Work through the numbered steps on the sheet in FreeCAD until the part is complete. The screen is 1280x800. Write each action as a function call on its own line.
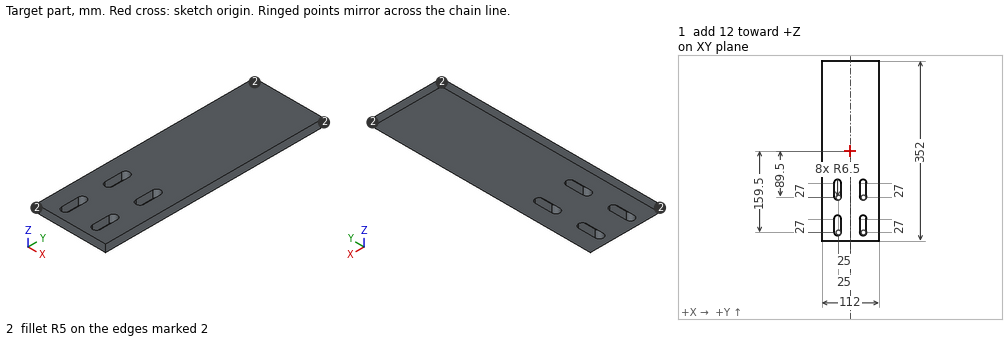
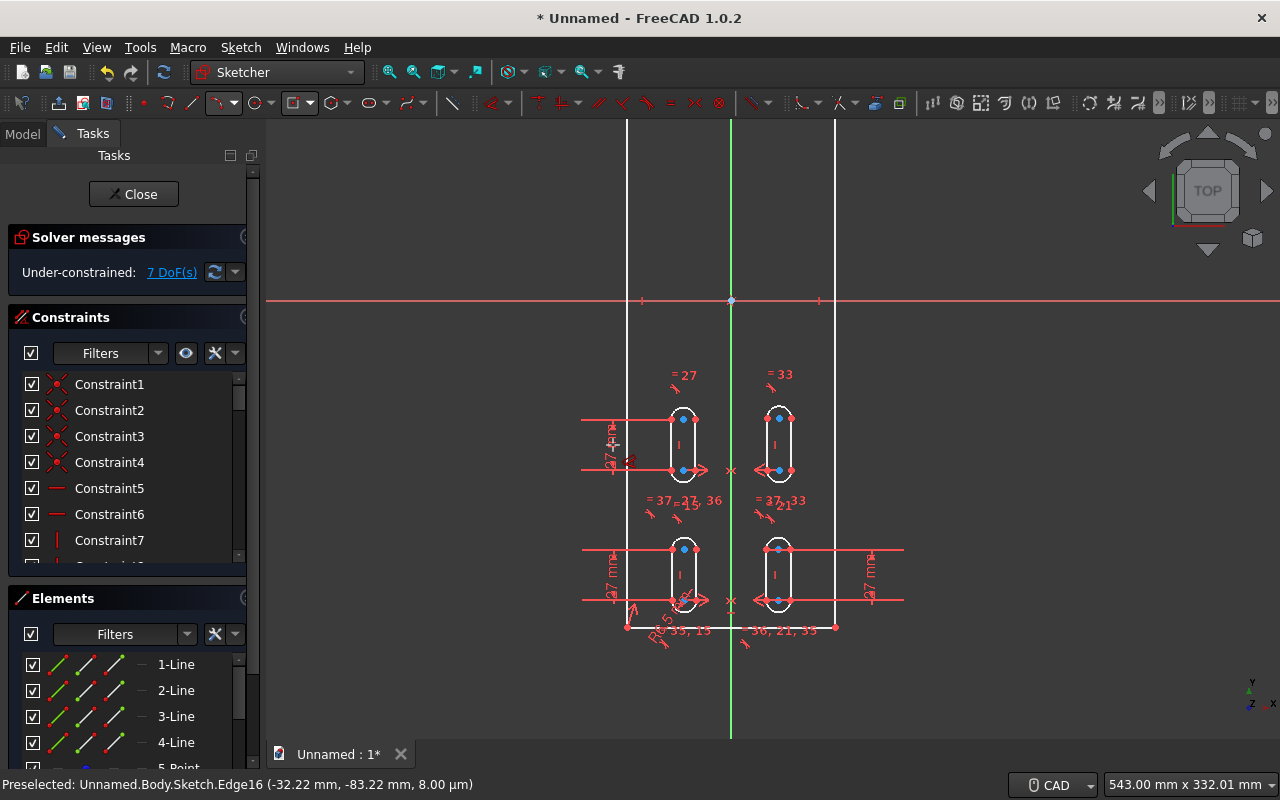
click(767, 455)
click(709, 444)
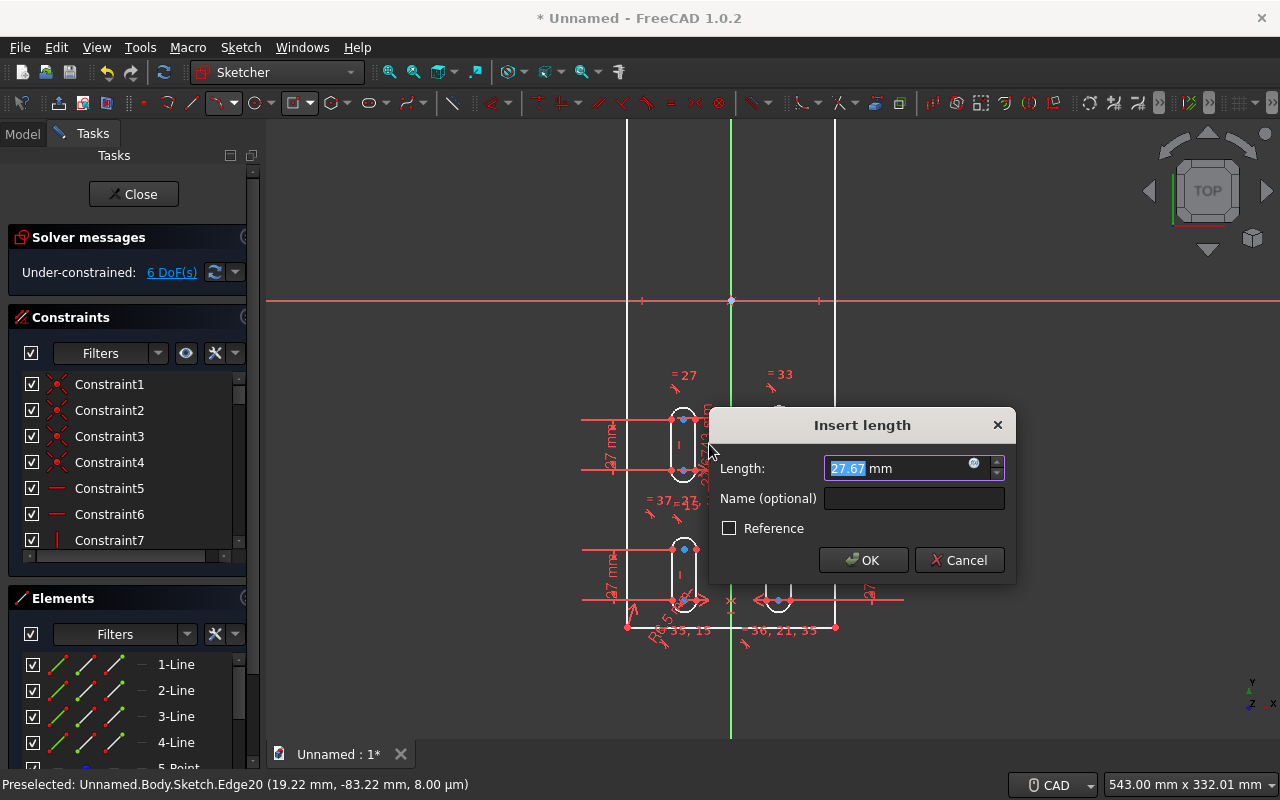
text(27)
key(Return)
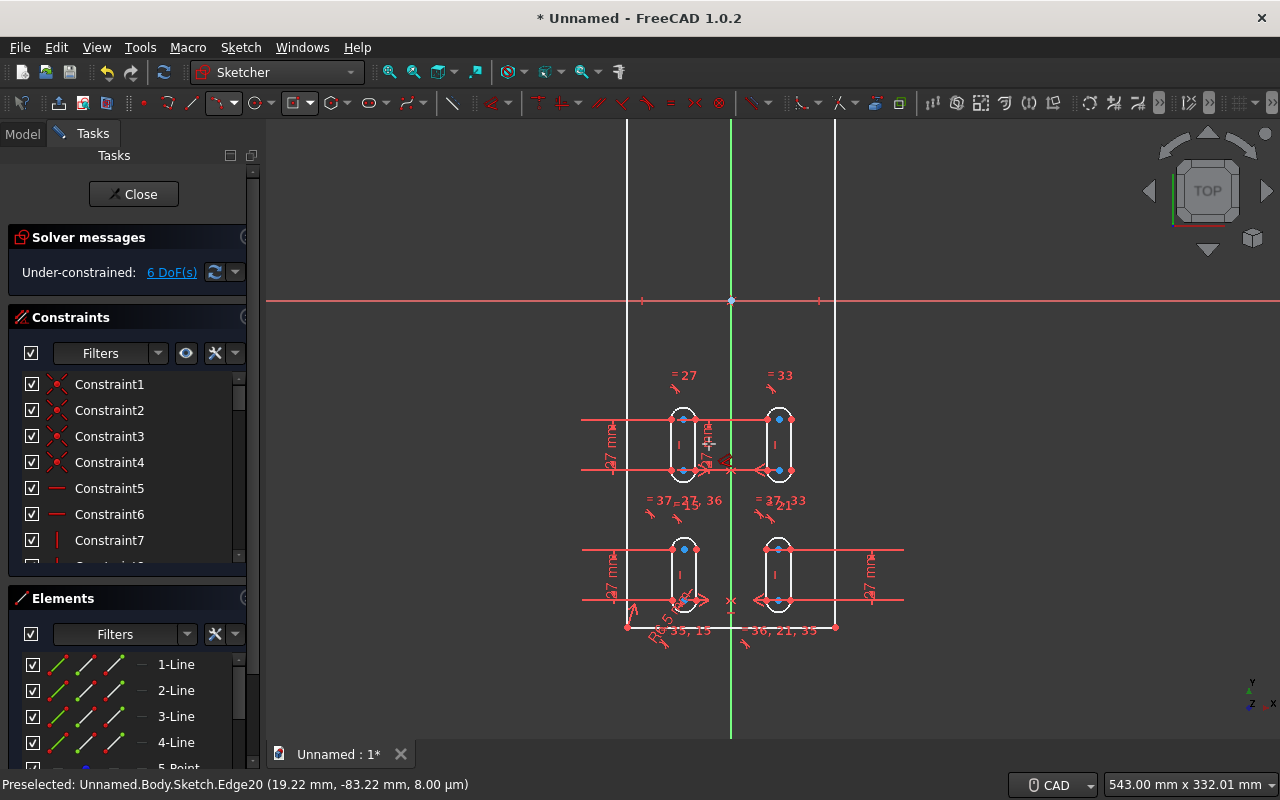
click(690, 628)
click(683, 662)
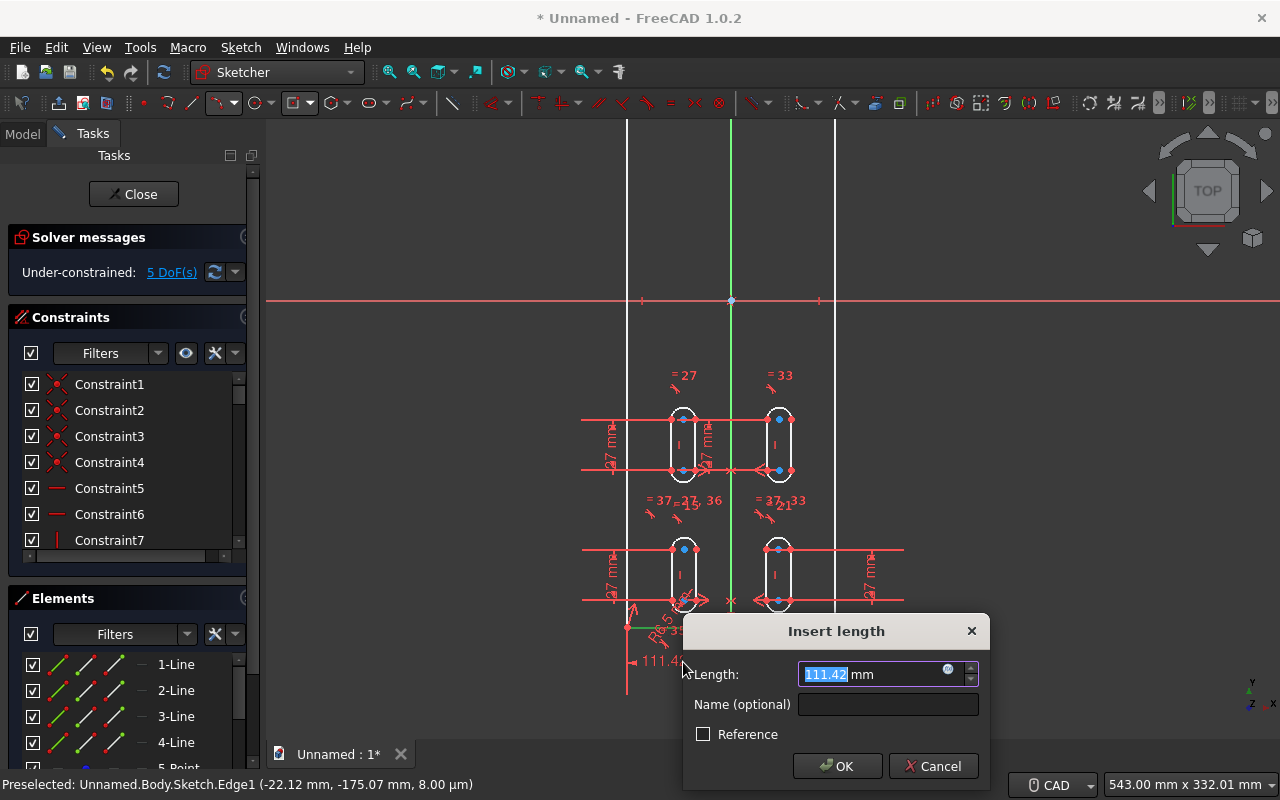
text(112)
key(Return)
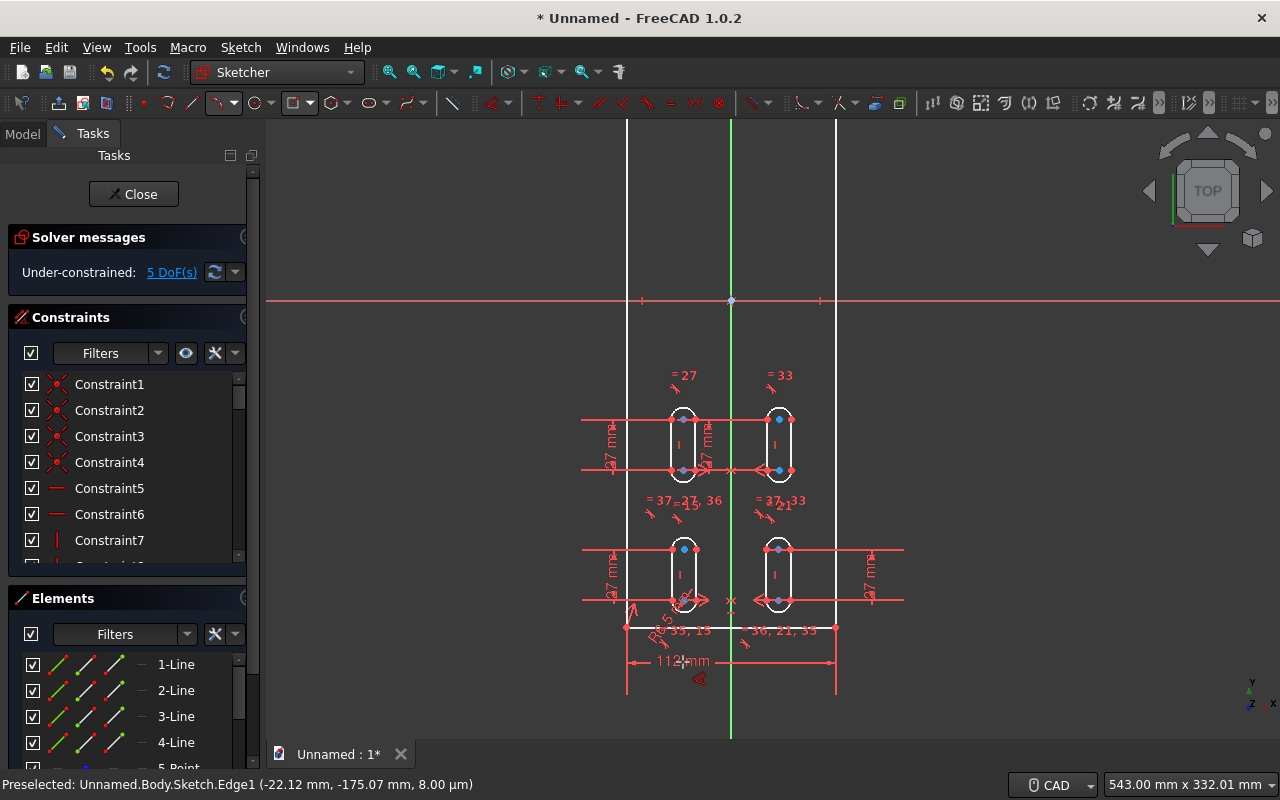
click(836, 431)
click(870, 387)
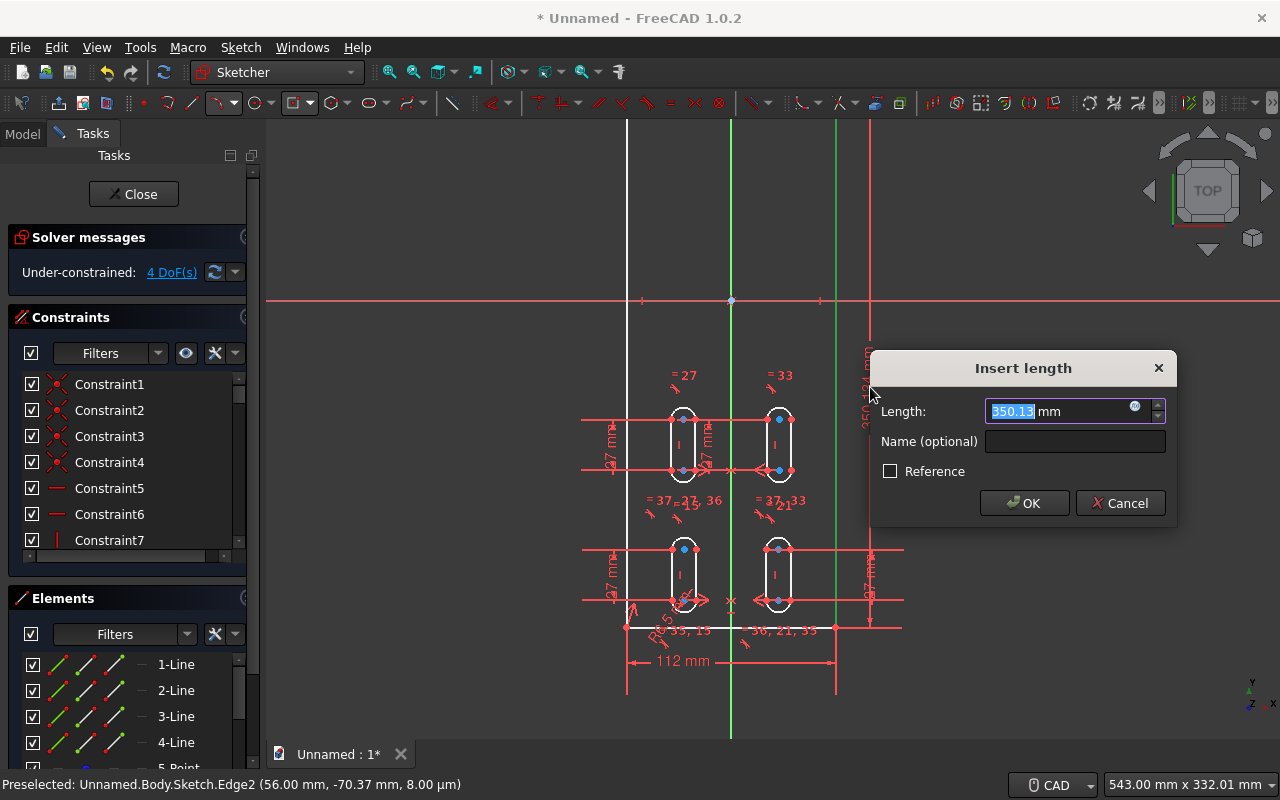
text(352)
key(Return)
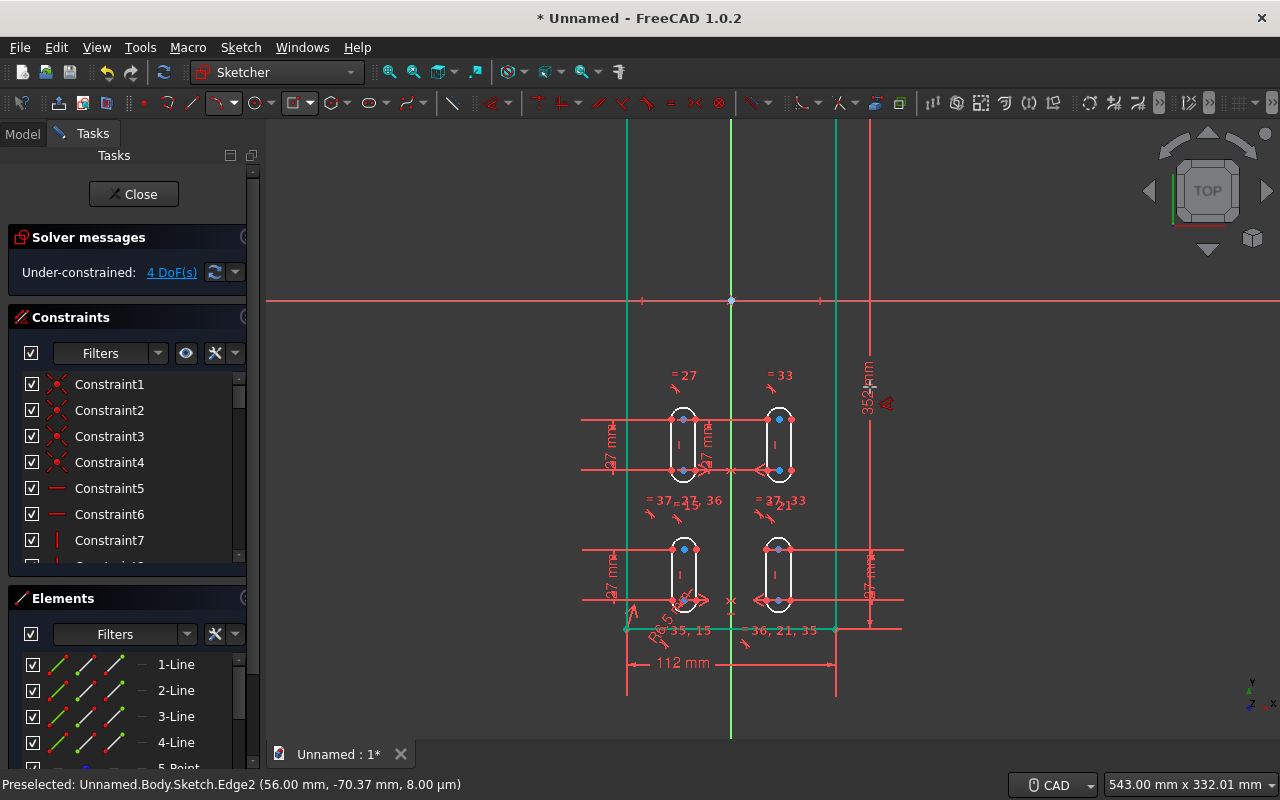
click(684, 600)
click(708, 267)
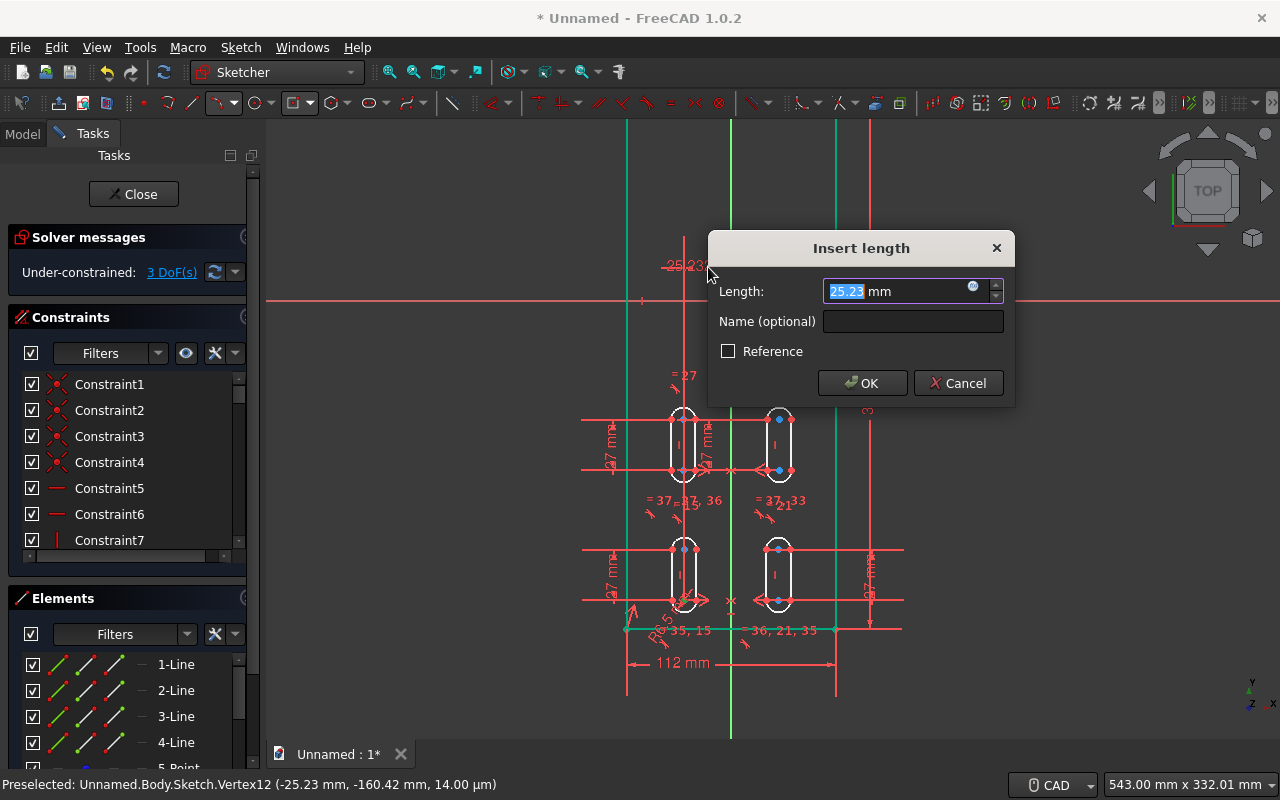
text(25)
key(Return)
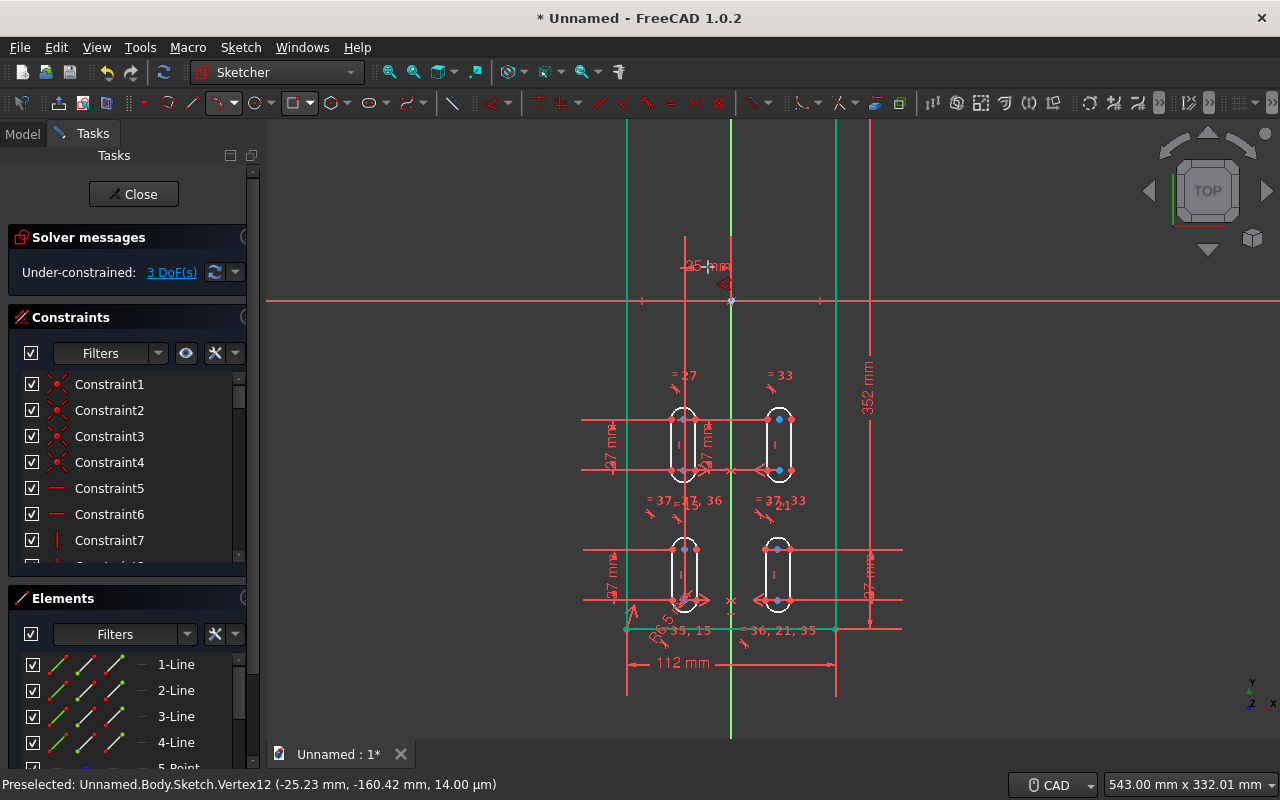
click(683, 470)
click(707, 504)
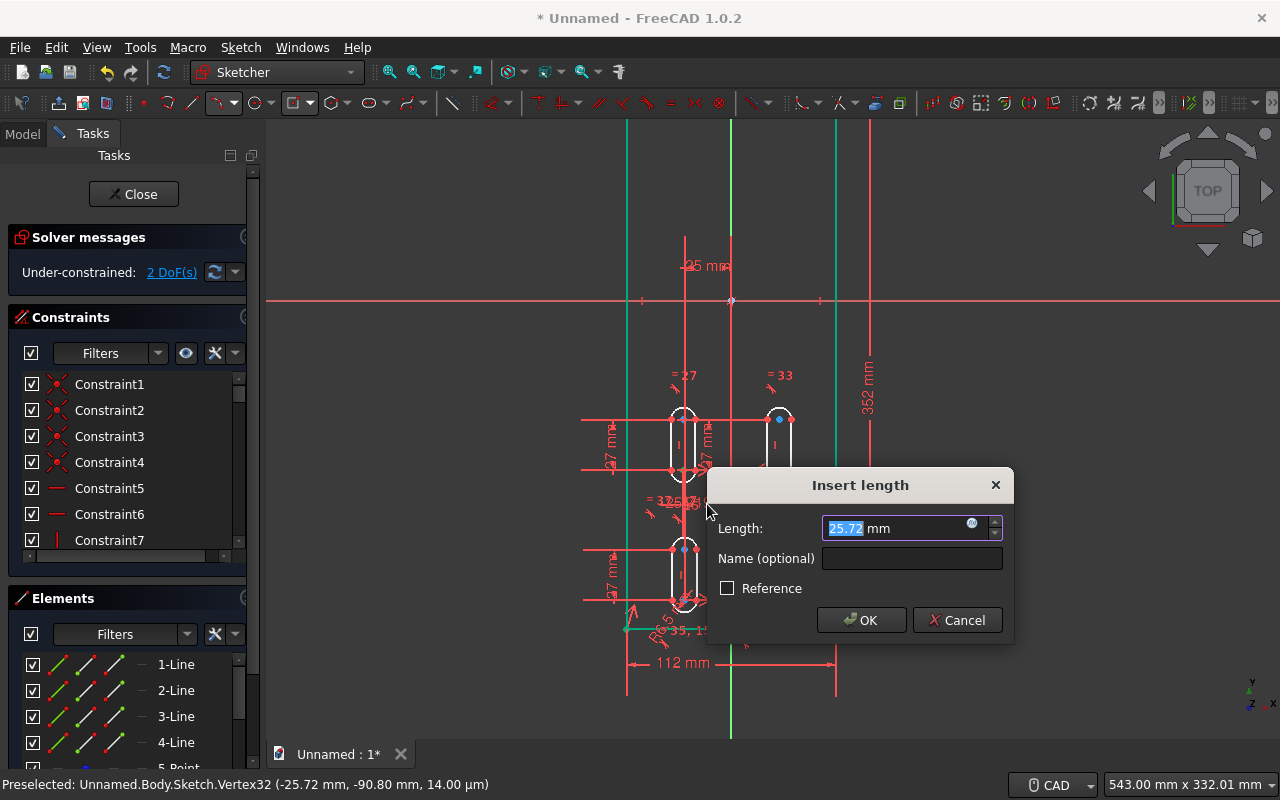
text(25)
key(Return)